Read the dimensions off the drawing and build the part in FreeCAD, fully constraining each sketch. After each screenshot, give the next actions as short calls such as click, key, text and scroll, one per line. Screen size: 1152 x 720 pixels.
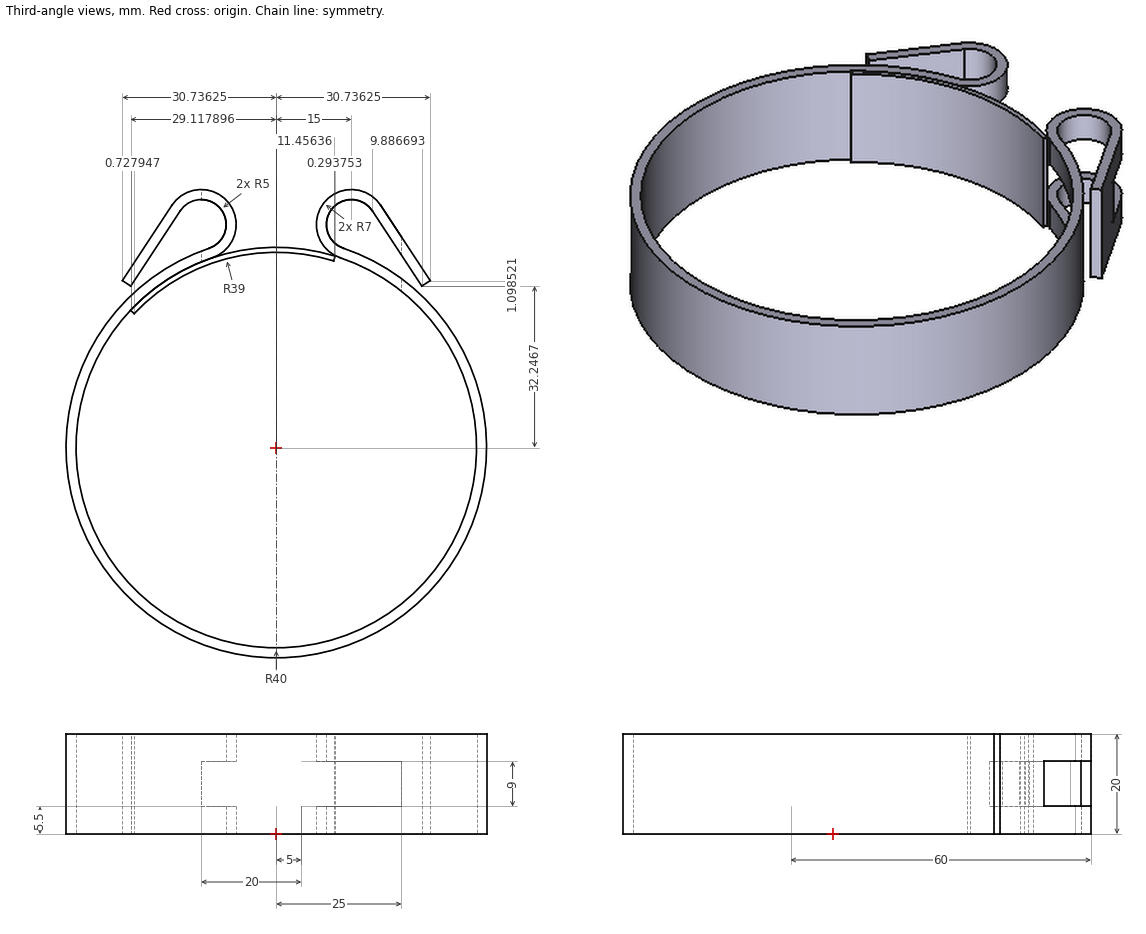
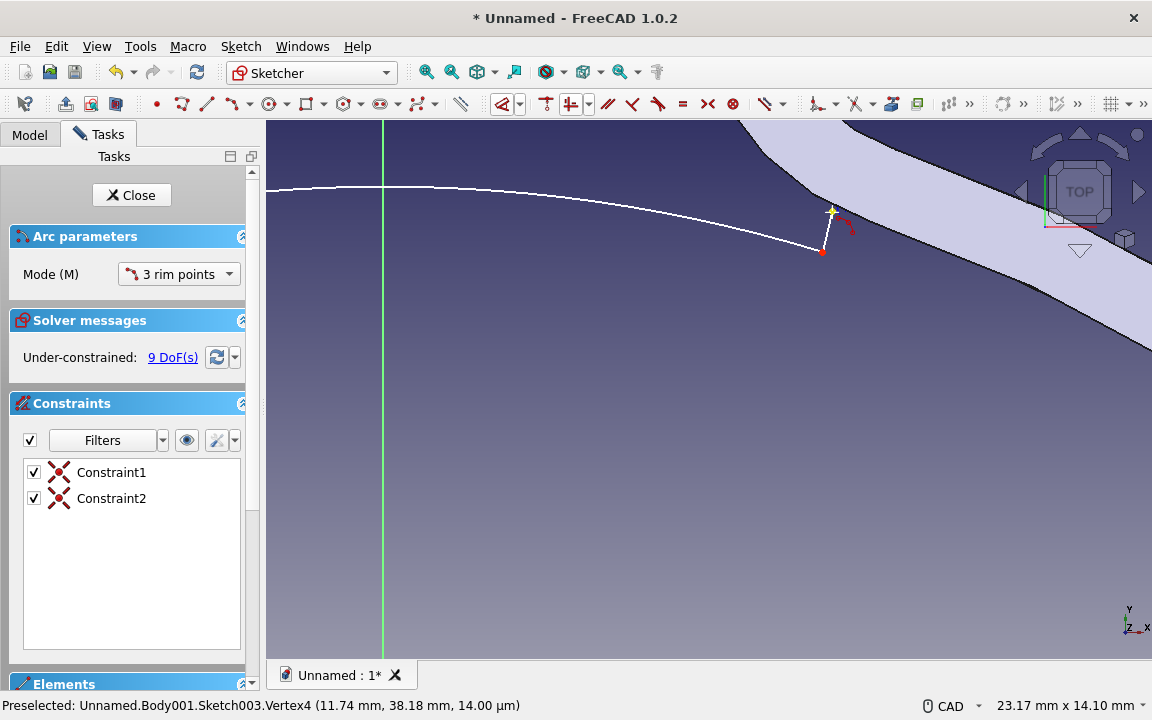
scroll(833, 212, down, 7)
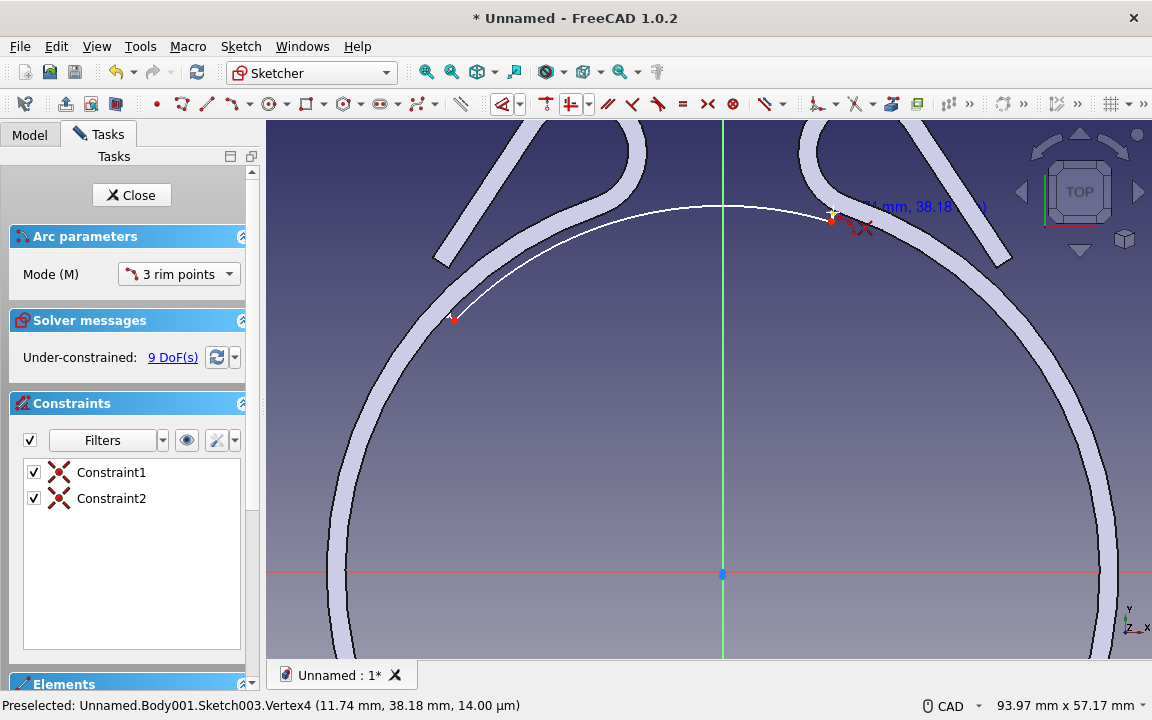
scroll(448, 313, up, 7)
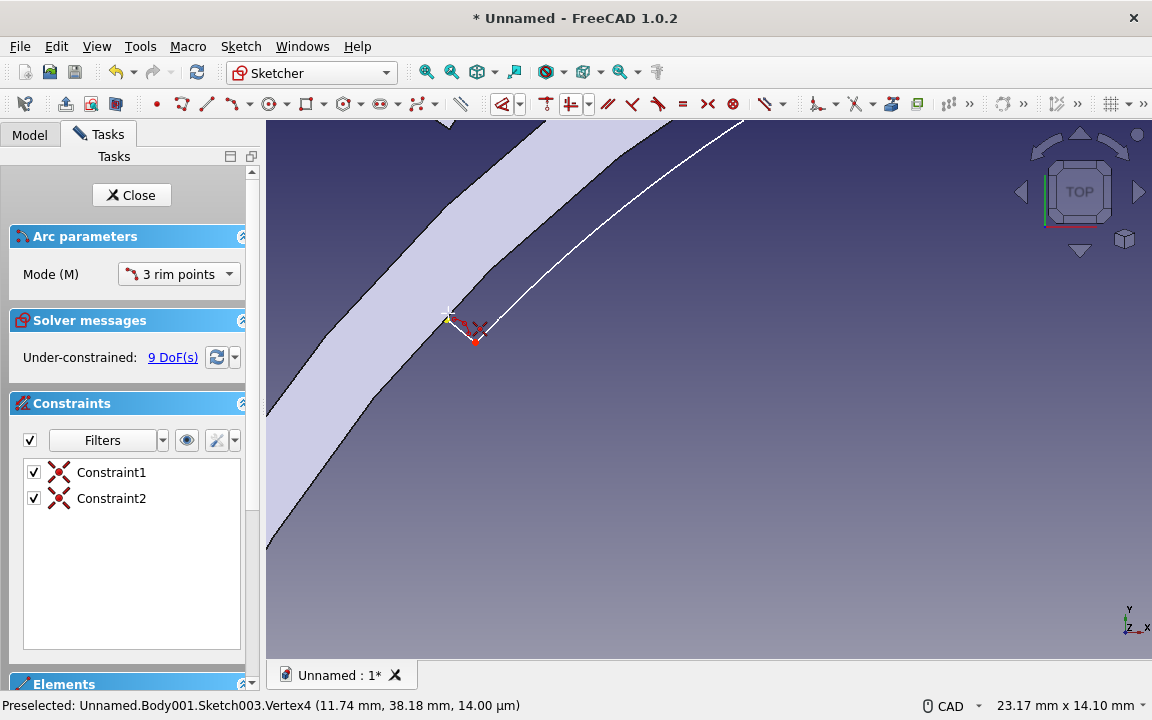
click(447, 320)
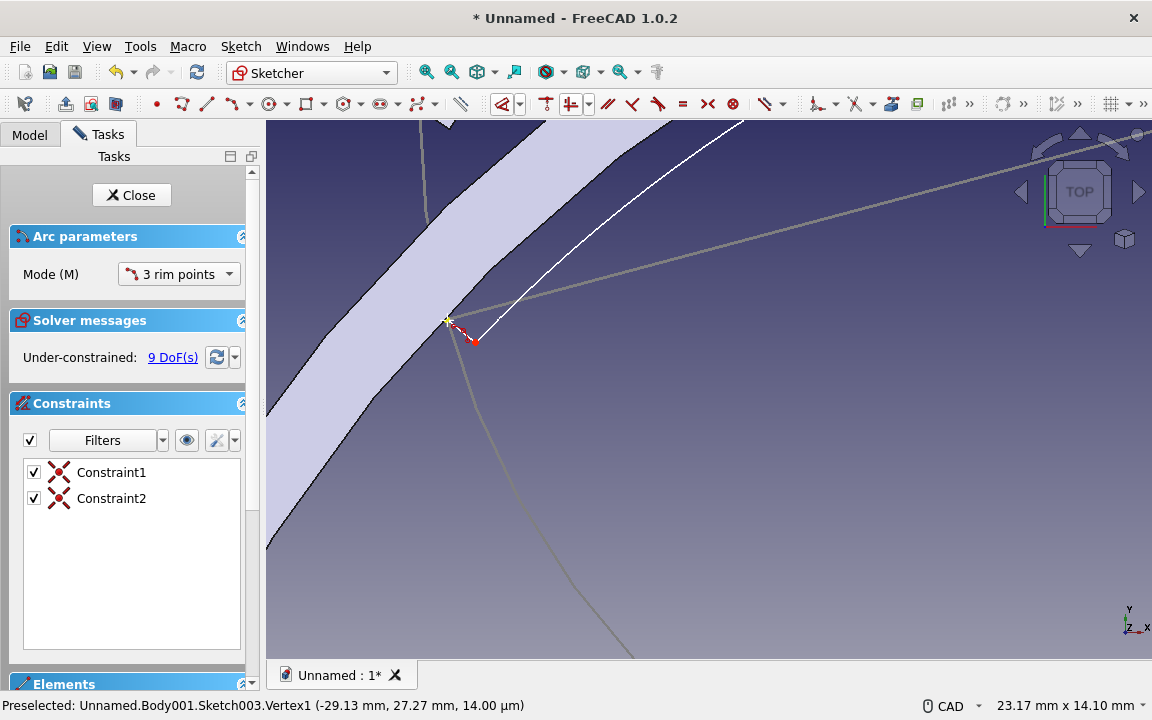
scroll(448, 313, down, 7)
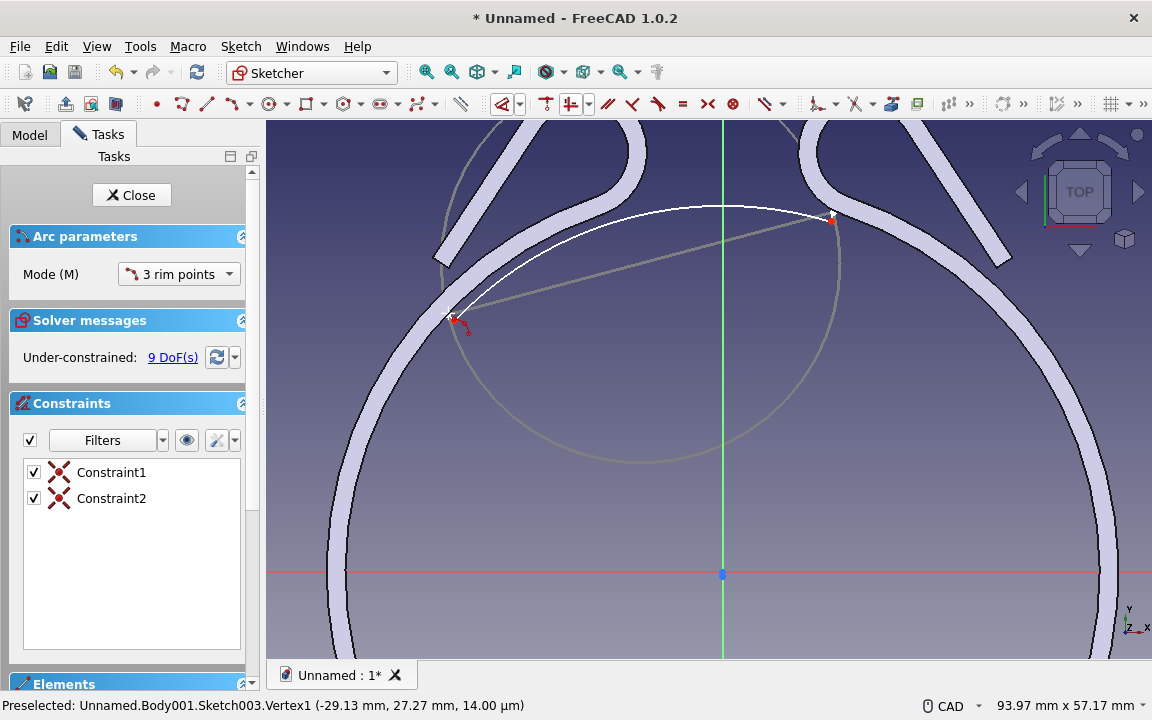
scroll(626, 207, up, 3)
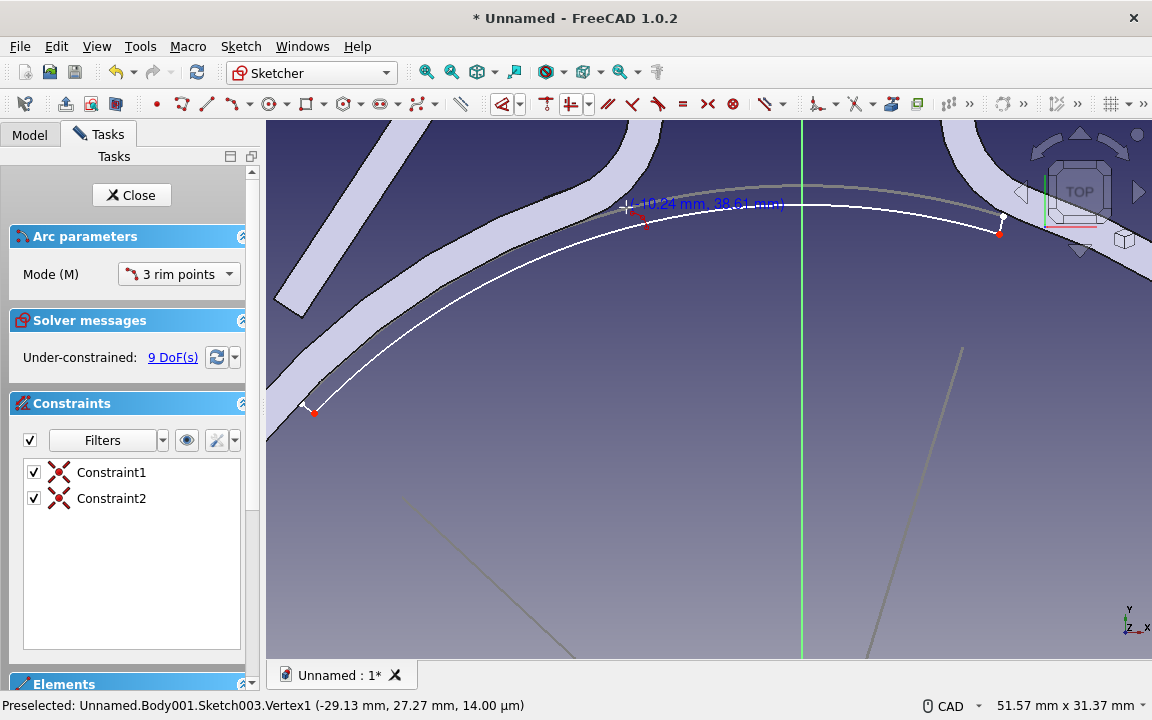
click(626, 208)
key(Escape)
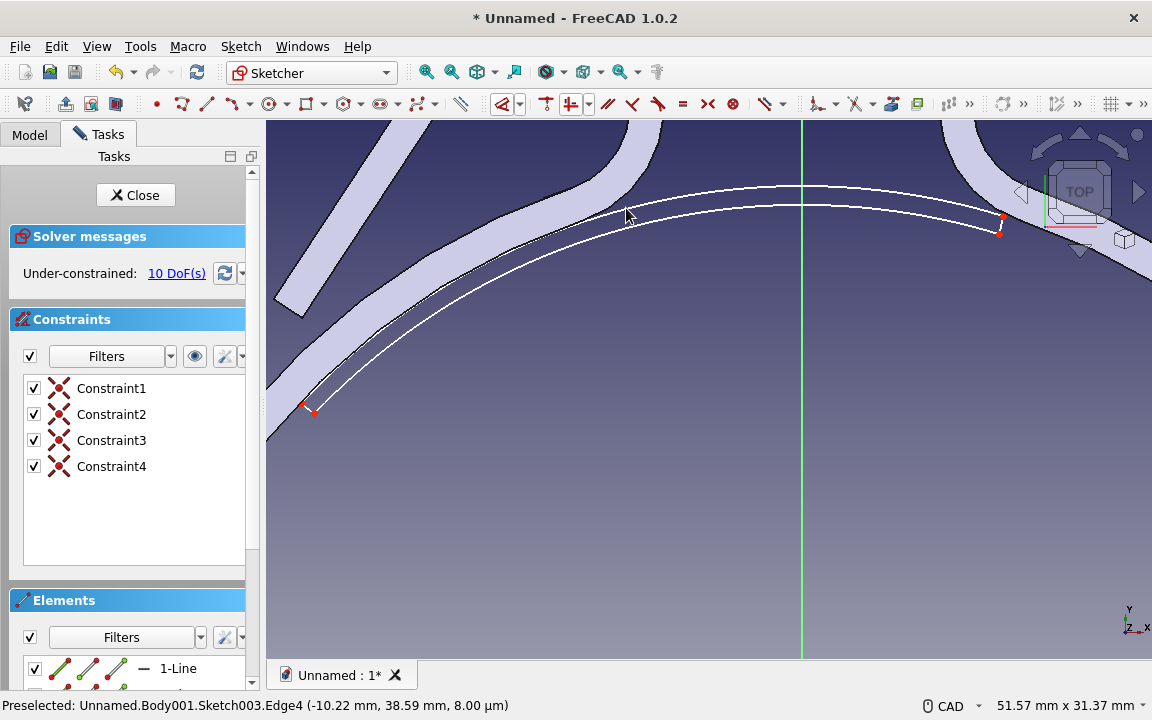
click(778, 205)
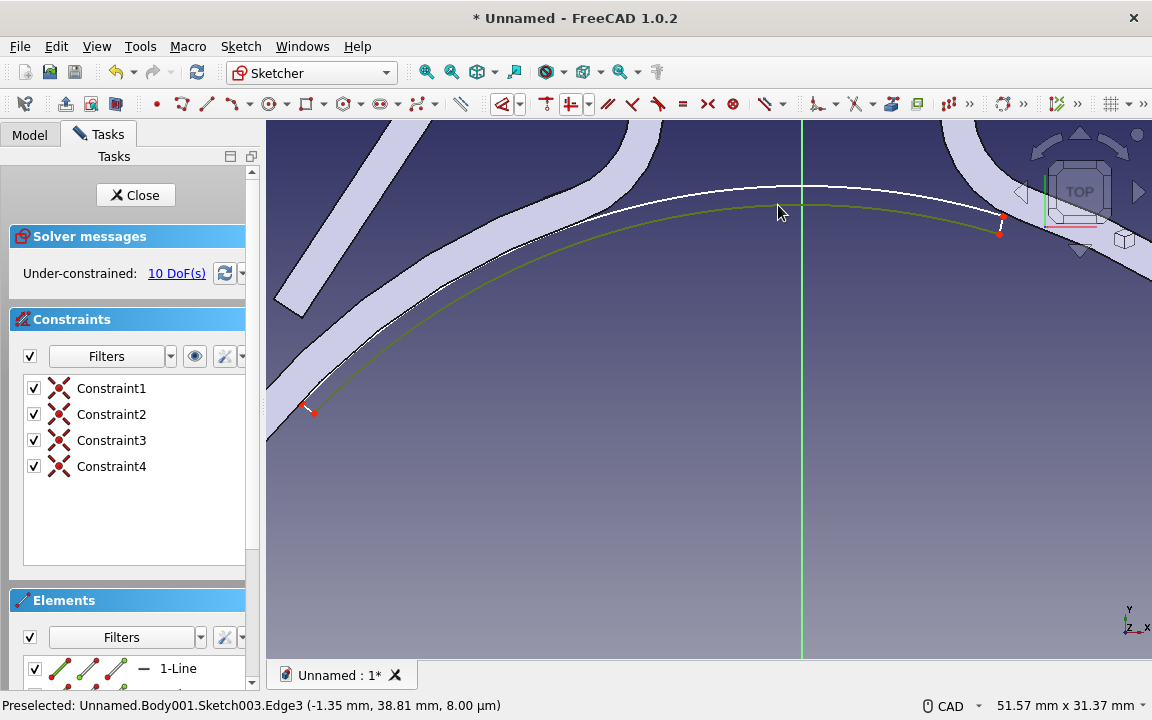
click(777, 186)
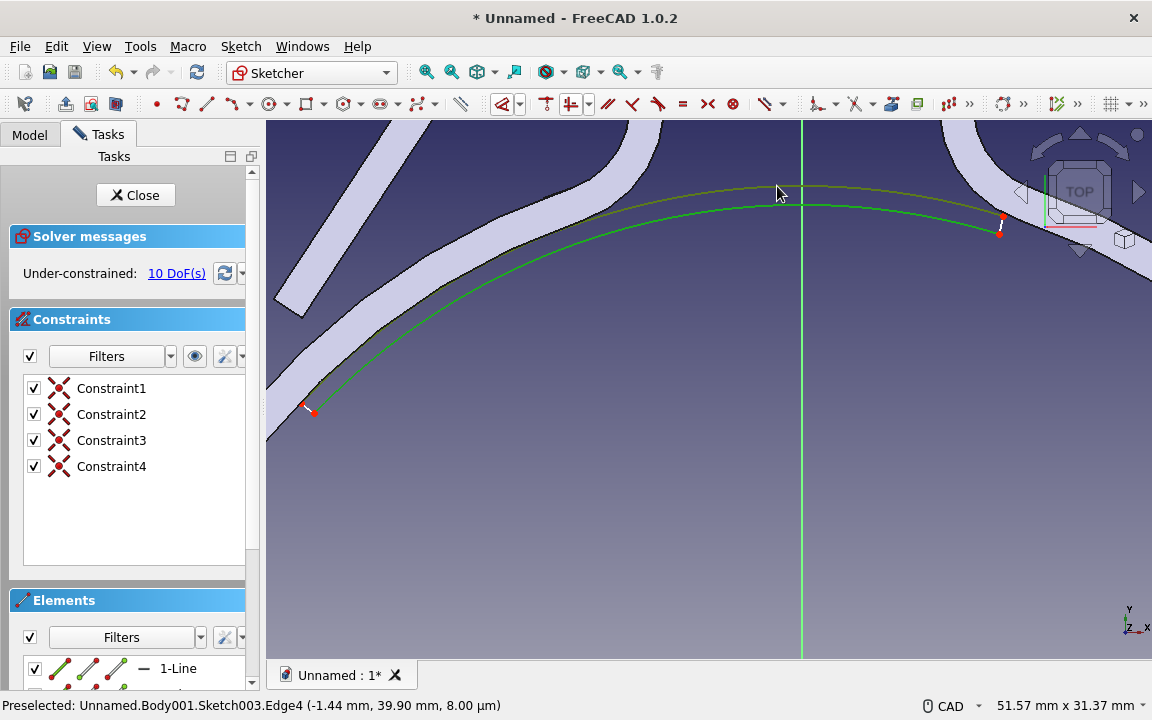
click(546, 104)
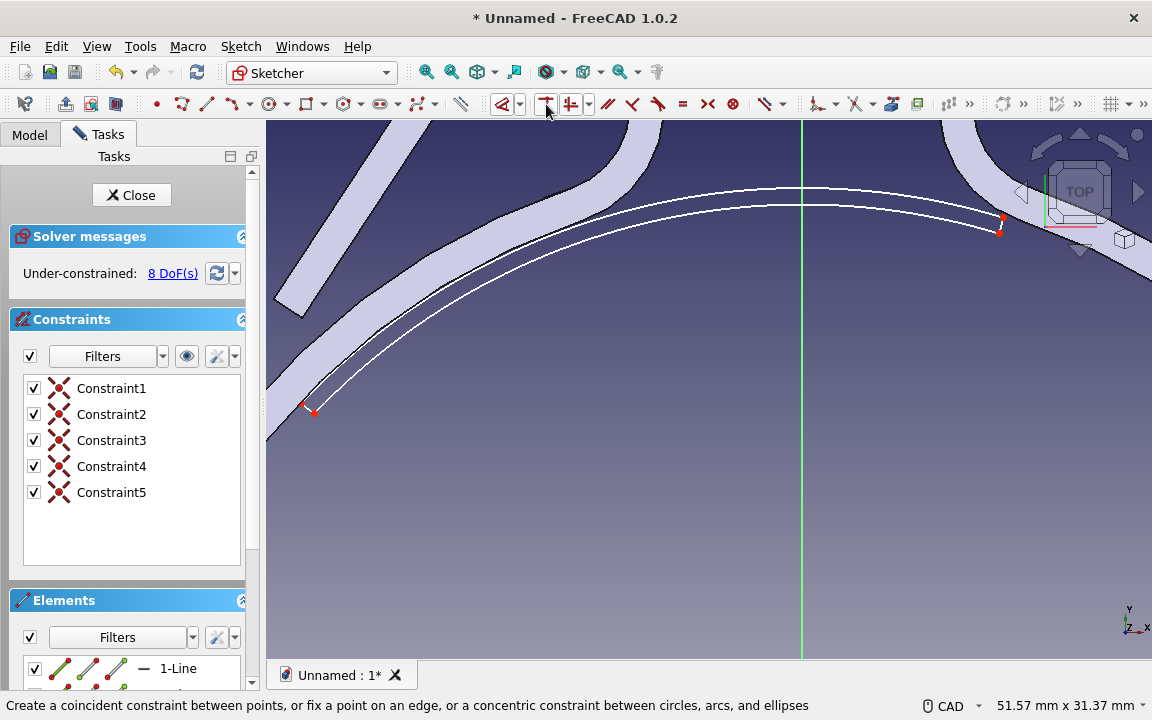
scroll(626, 207, down, 3)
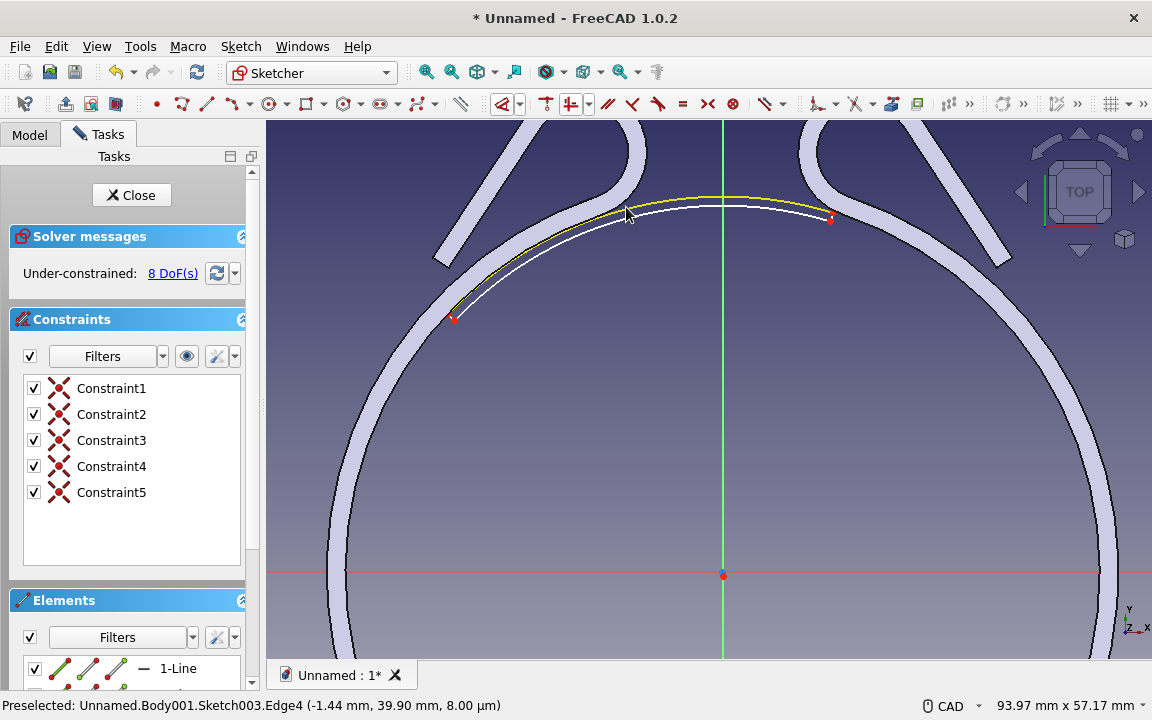
drag(713, 562, 733, 586)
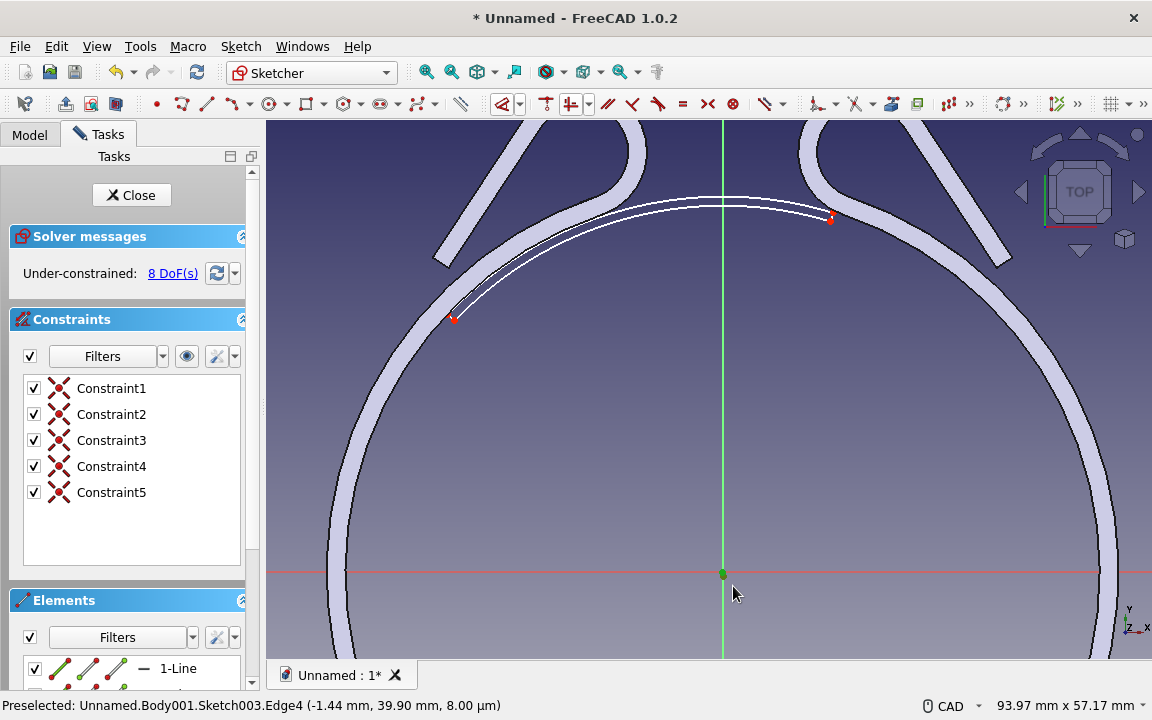
key(c)